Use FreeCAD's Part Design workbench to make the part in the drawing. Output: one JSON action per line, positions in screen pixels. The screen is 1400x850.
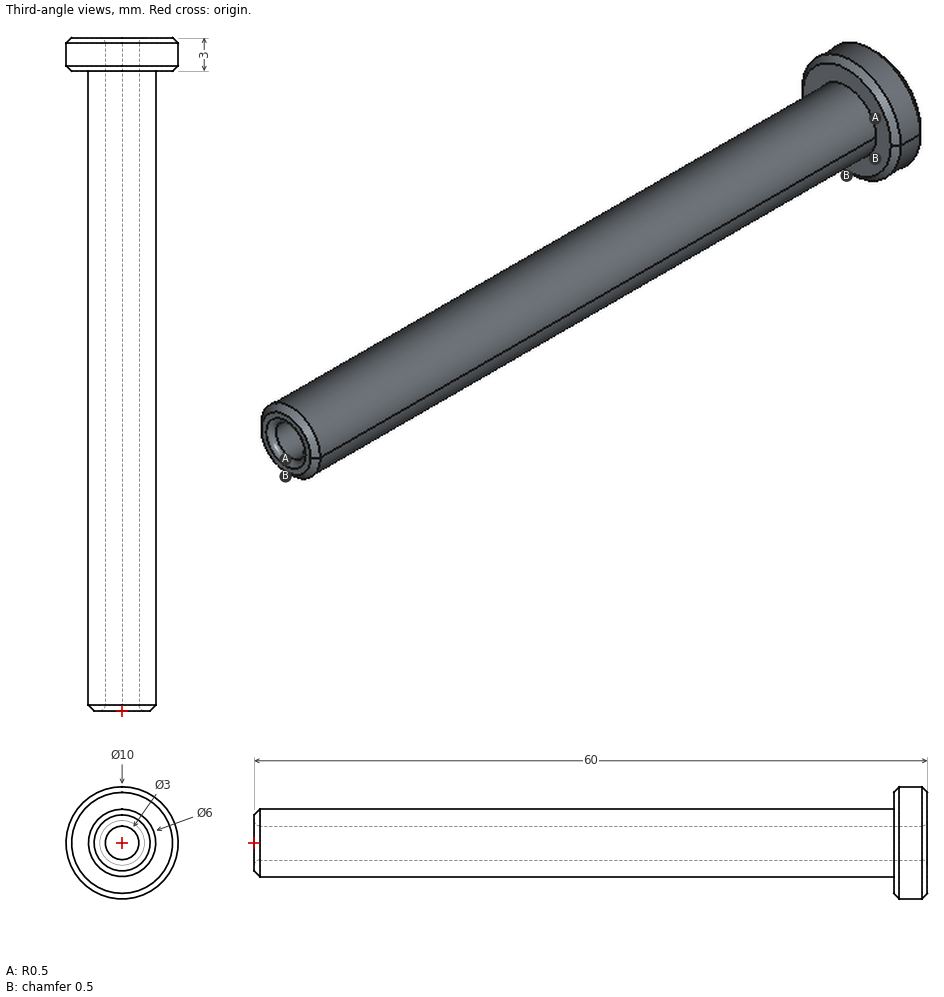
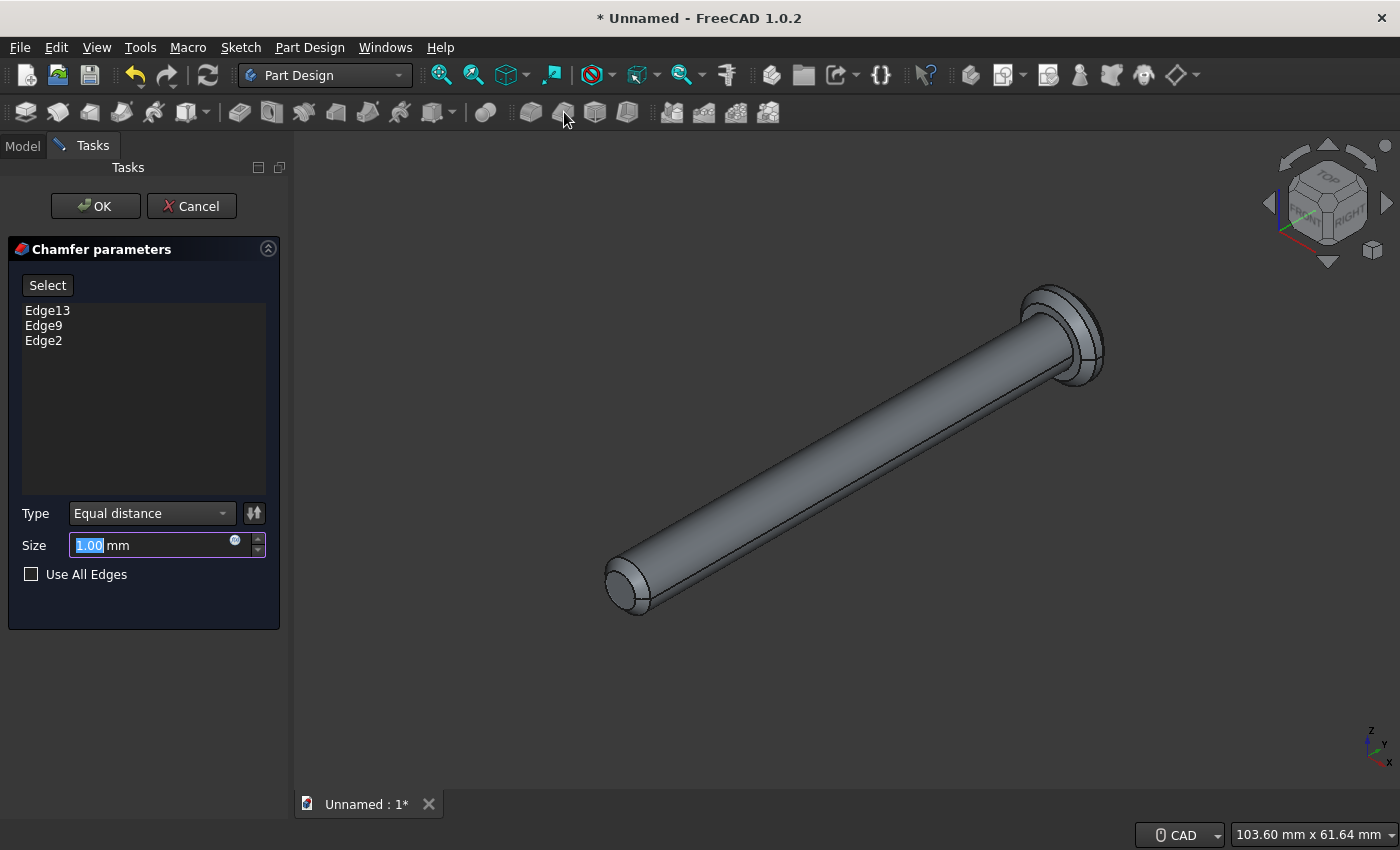
{"action": "type", "text": "0.5"}
{"action": "key", "text": "Tab"}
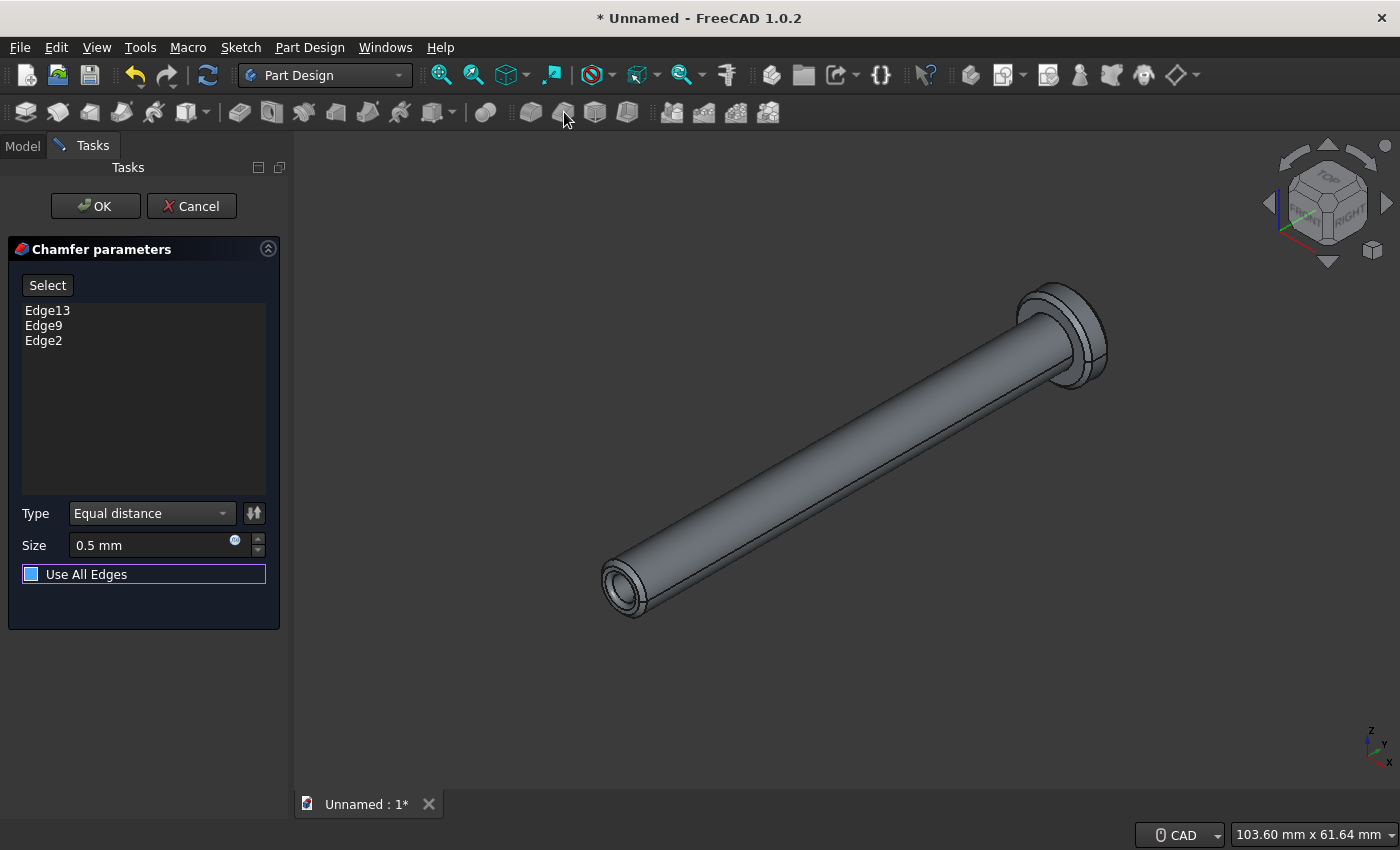
{"action": "left_click", "coordinate": [96, 206]}